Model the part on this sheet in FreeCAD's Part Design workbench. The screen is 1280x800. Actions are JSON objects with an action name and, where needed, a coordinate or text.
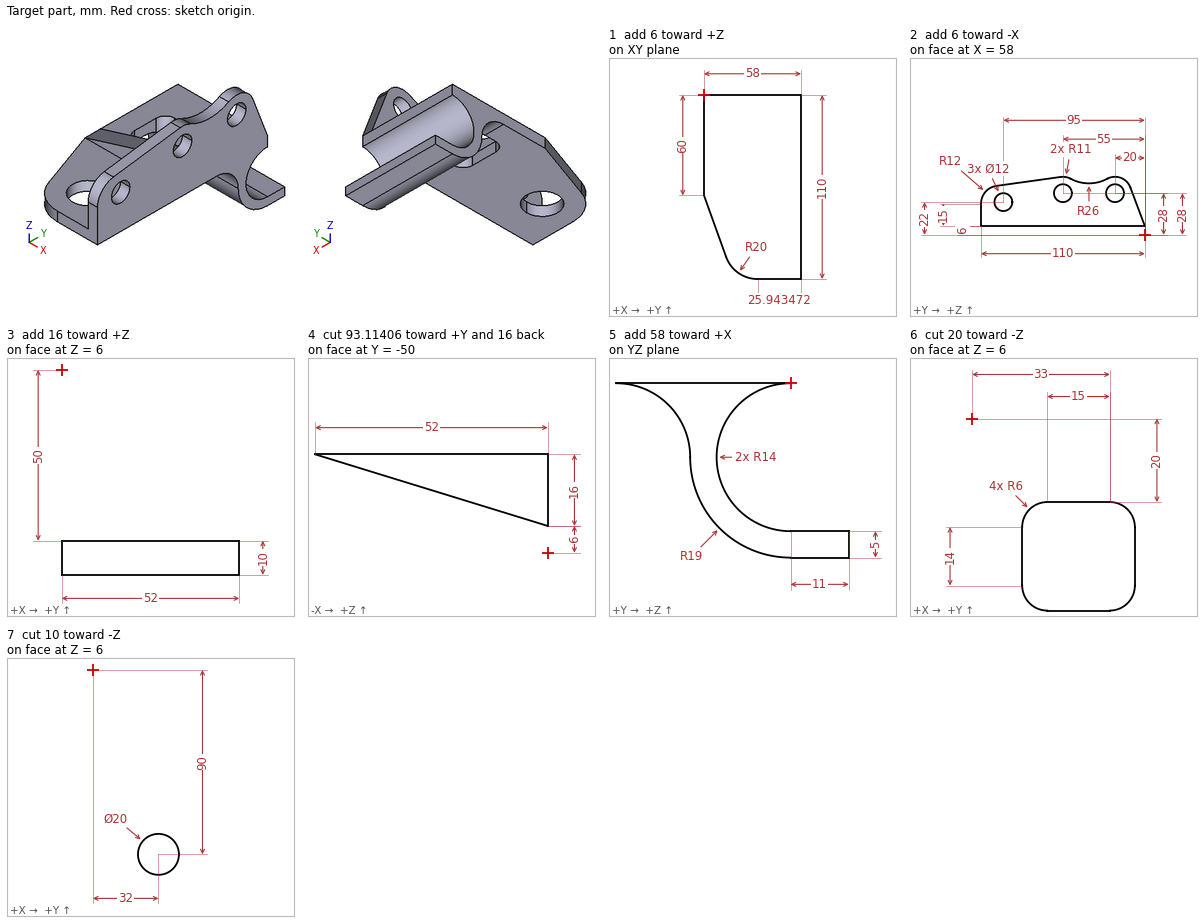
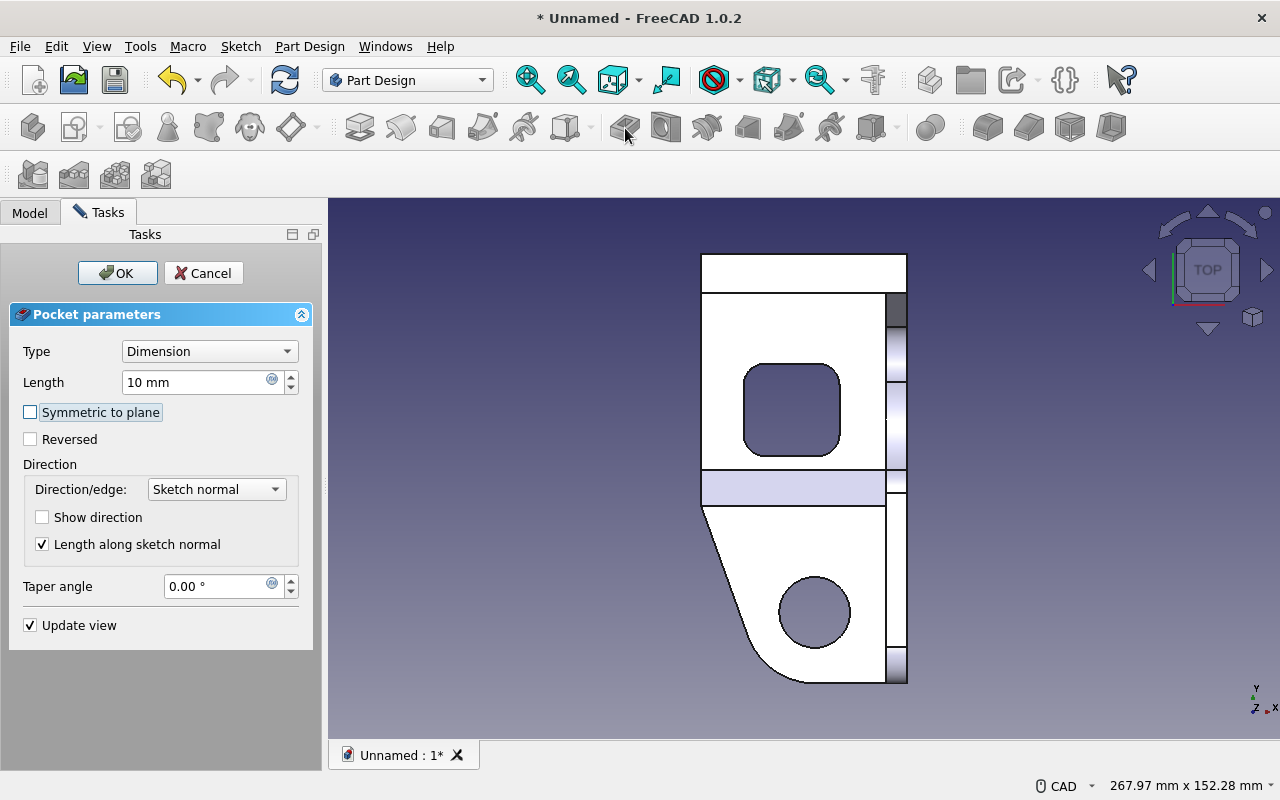
{"action": "left_click", "coordinate": [118, 273]}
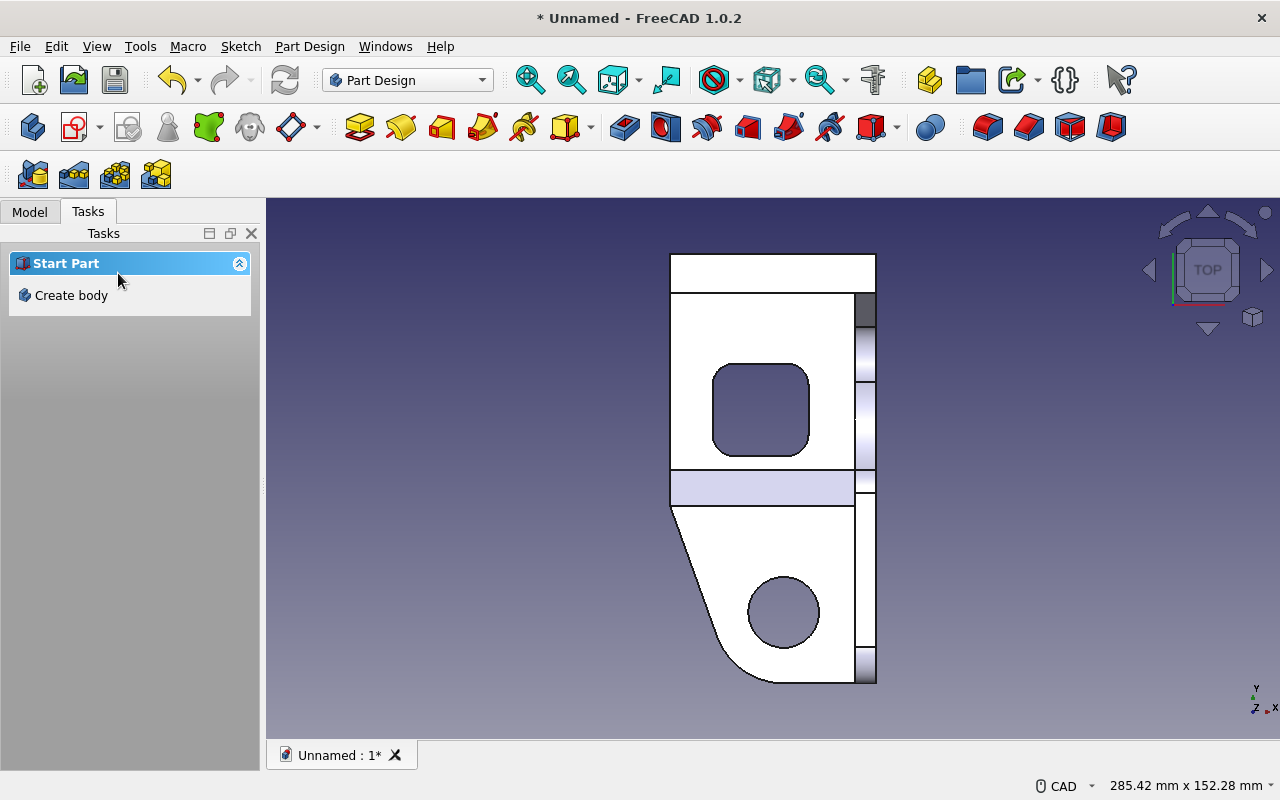
{"action": "key", "text": "0"}